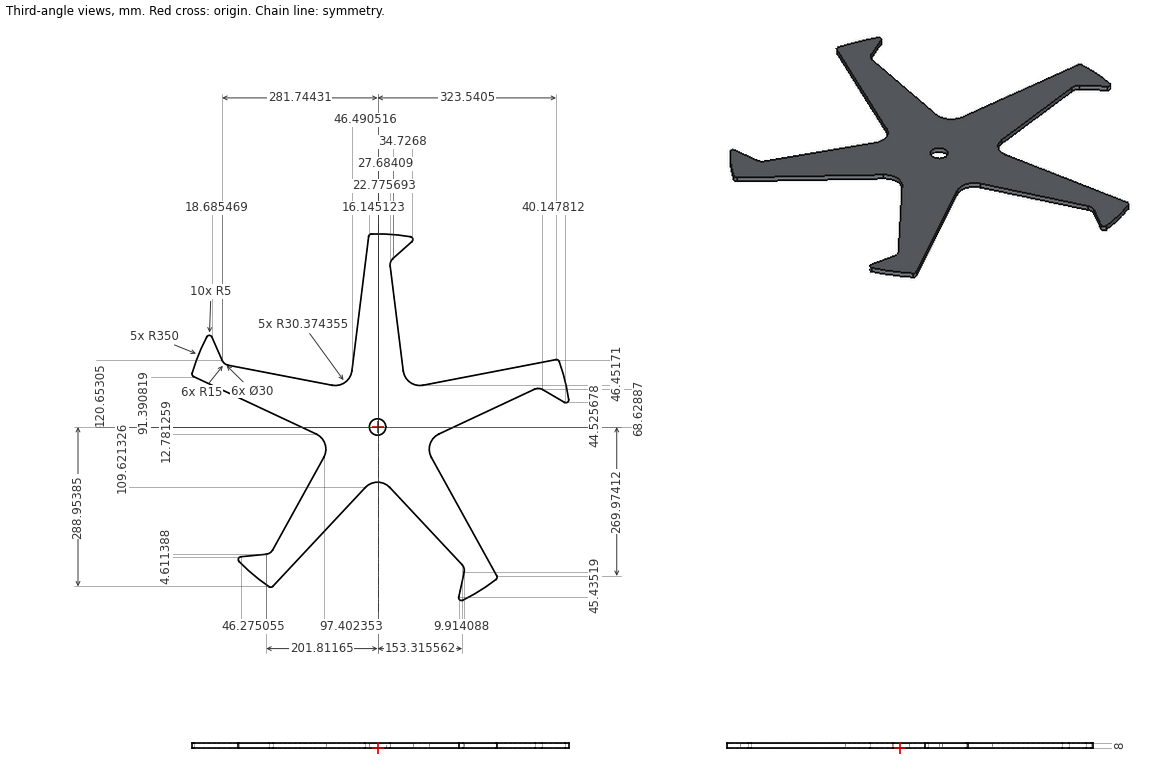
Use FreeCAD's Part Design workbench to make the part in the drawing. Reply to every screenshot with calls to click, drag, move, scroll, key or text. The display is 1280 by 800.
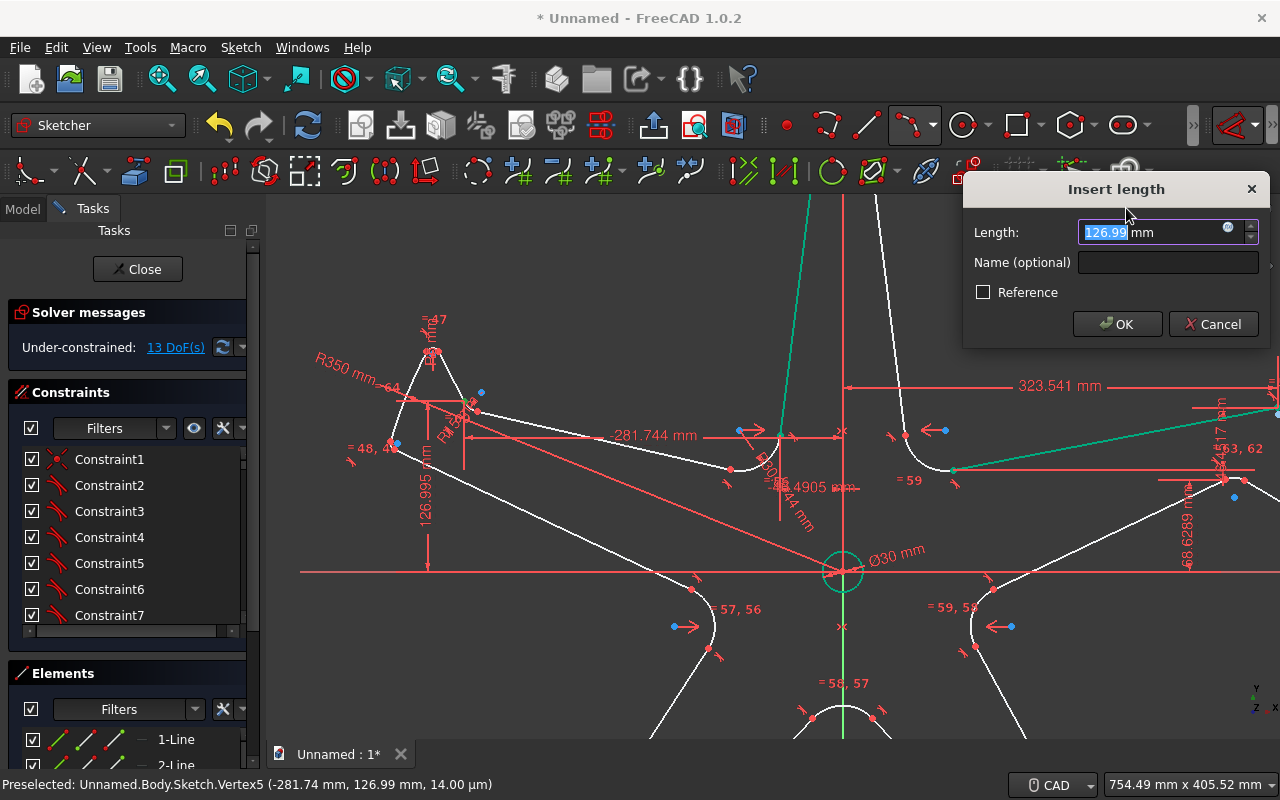
text(120.65305)
key(Return)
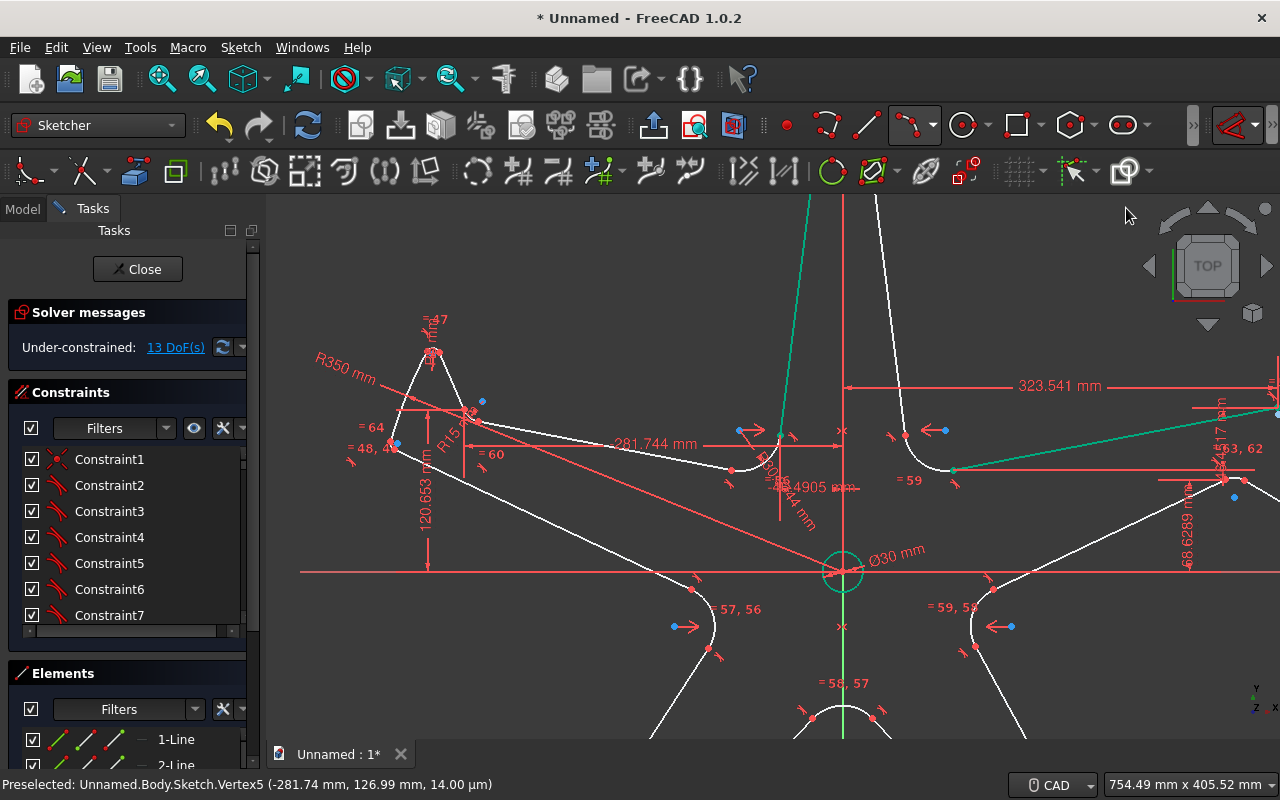
scroll(394, 449, up, 3)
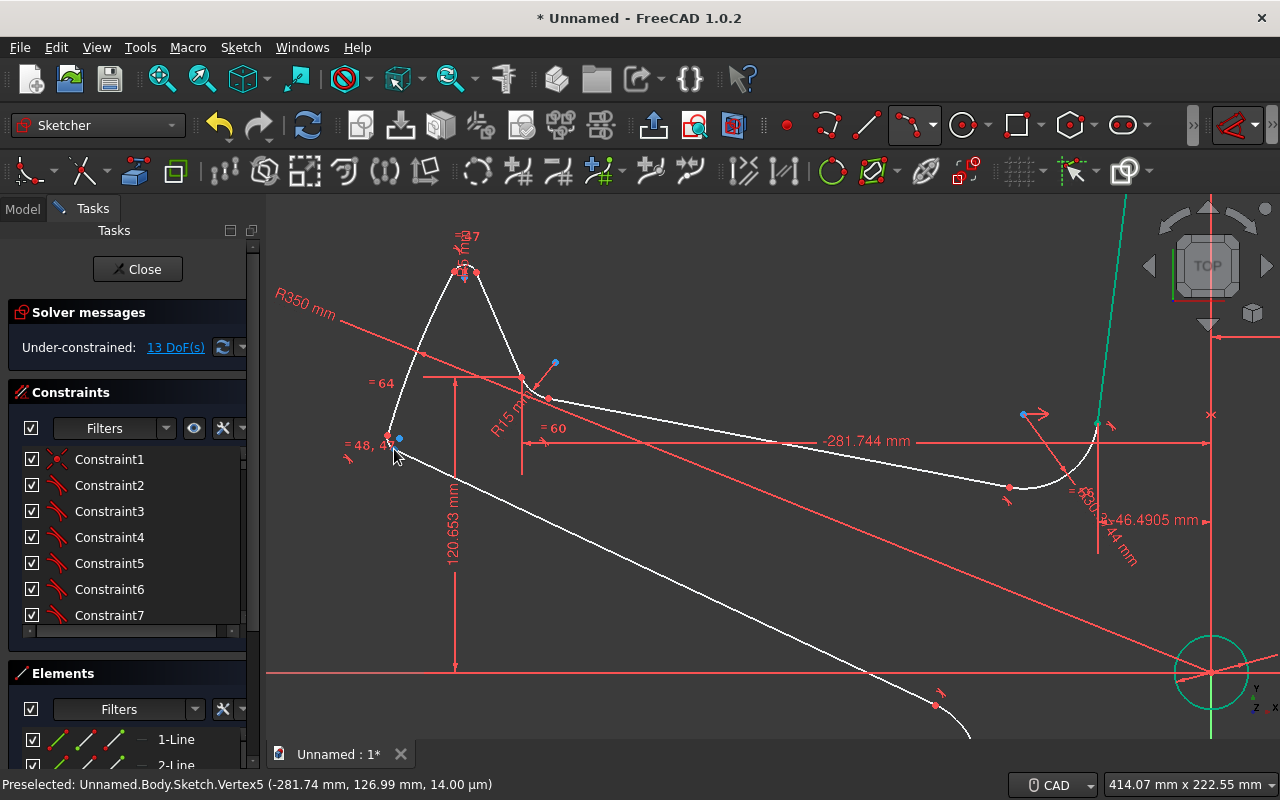
click(394, 449)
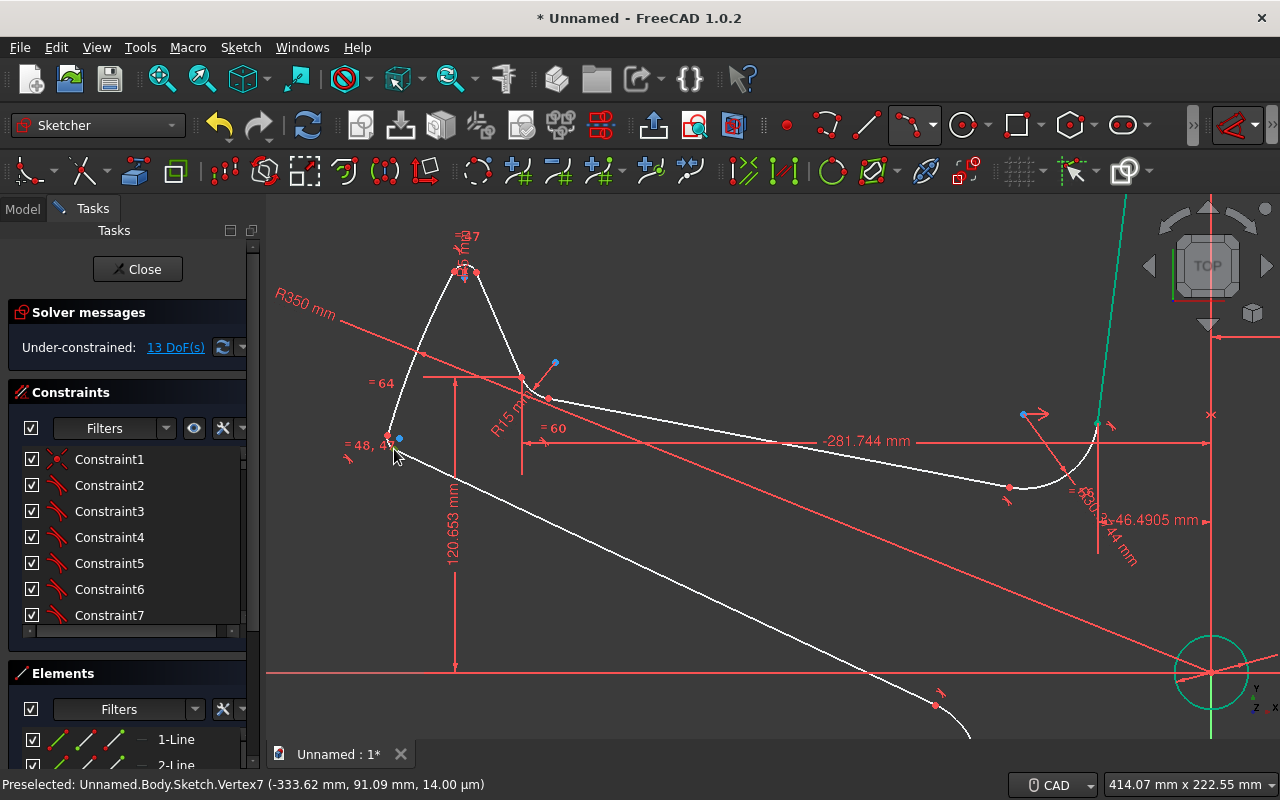
click(1258, 126)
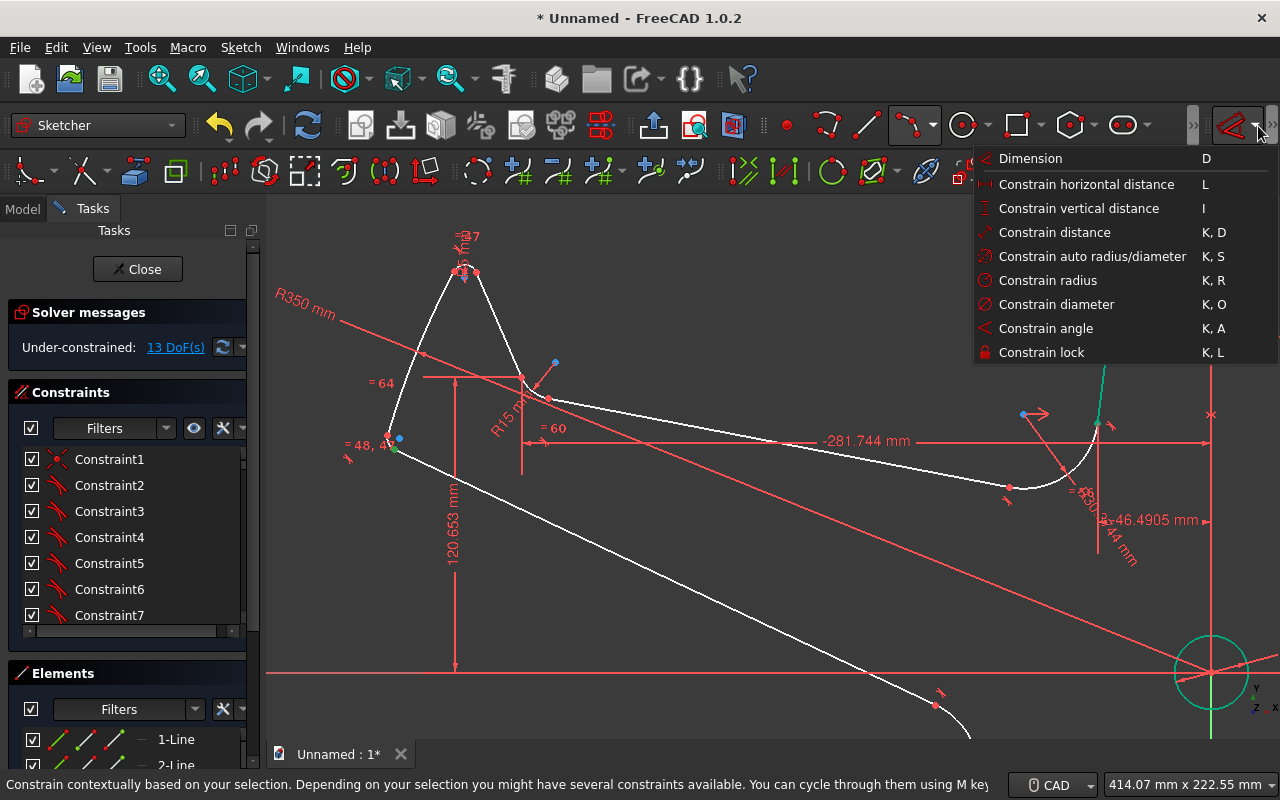
click(1126, 208)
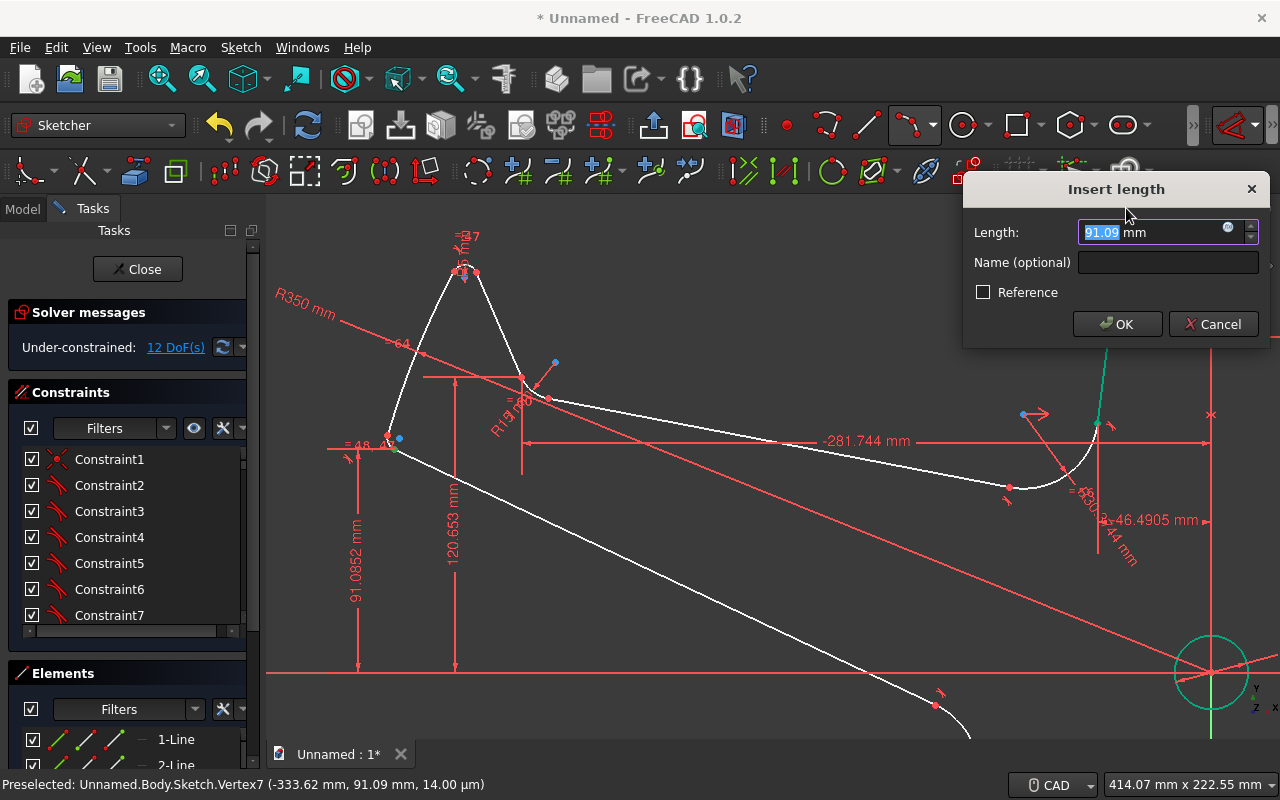
text(91.390819)
key(Return)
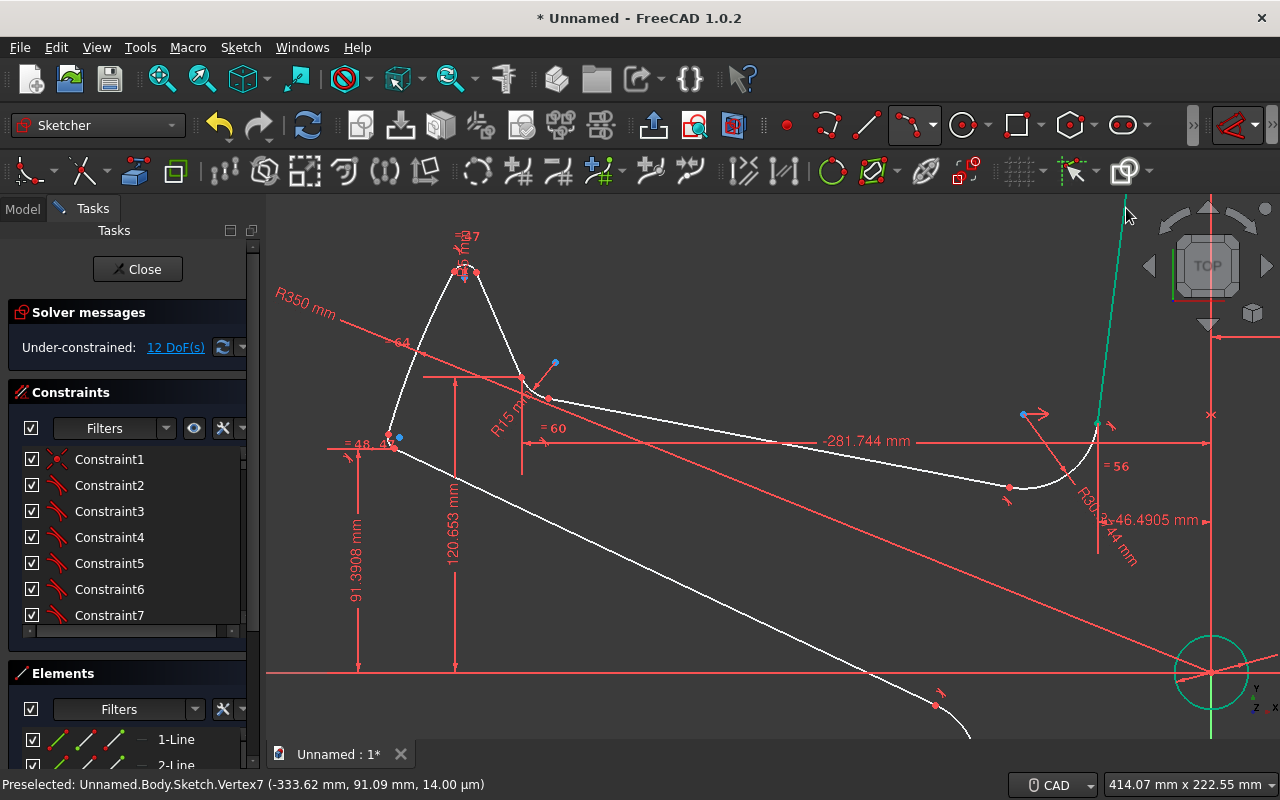
scroll(936, 705, up, 2)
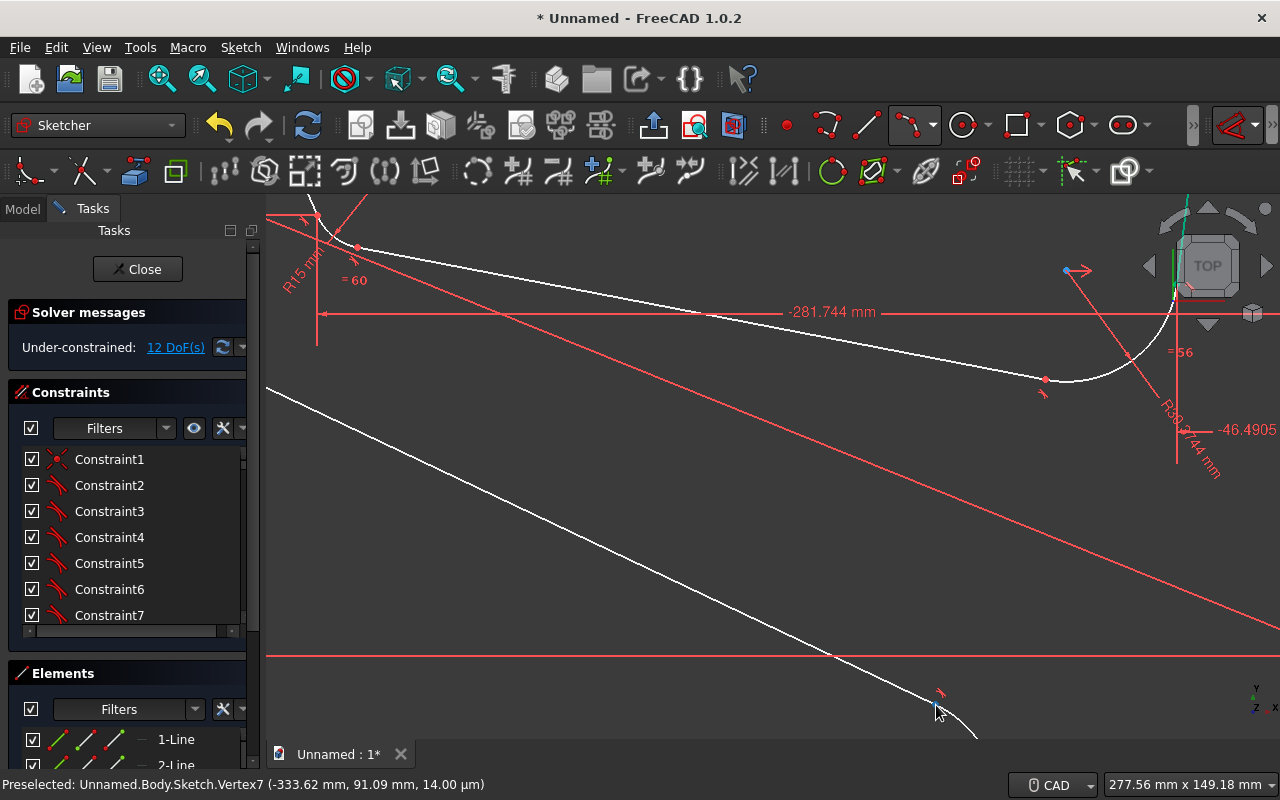
click(935, 705)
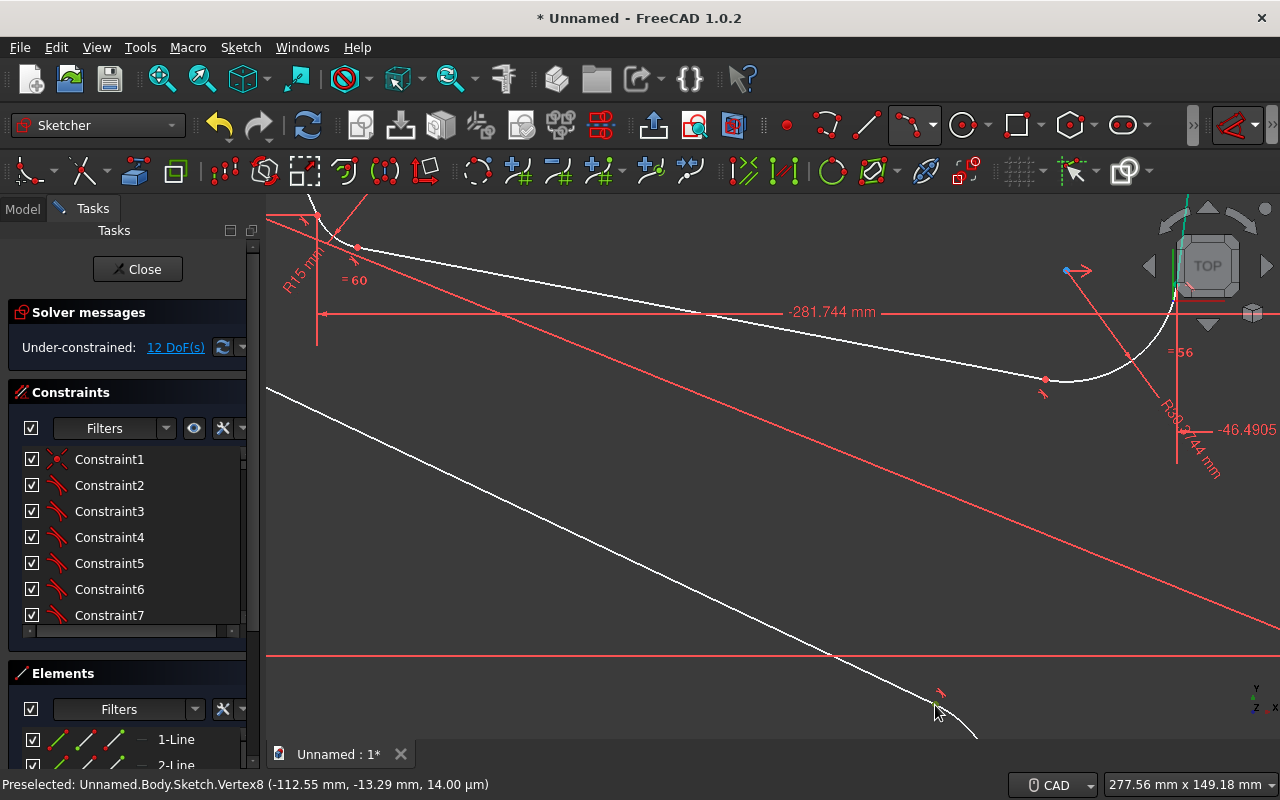
click(1258, 126)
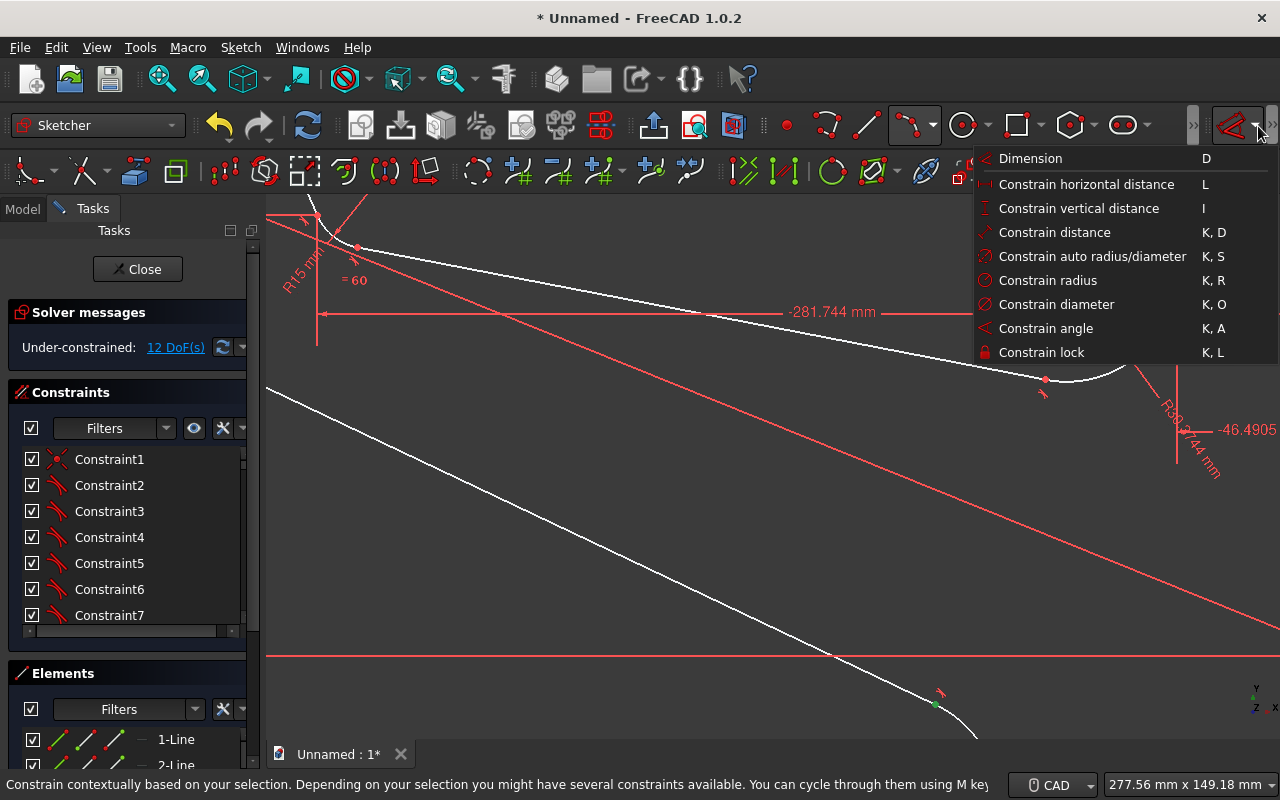
click(1126, 208)